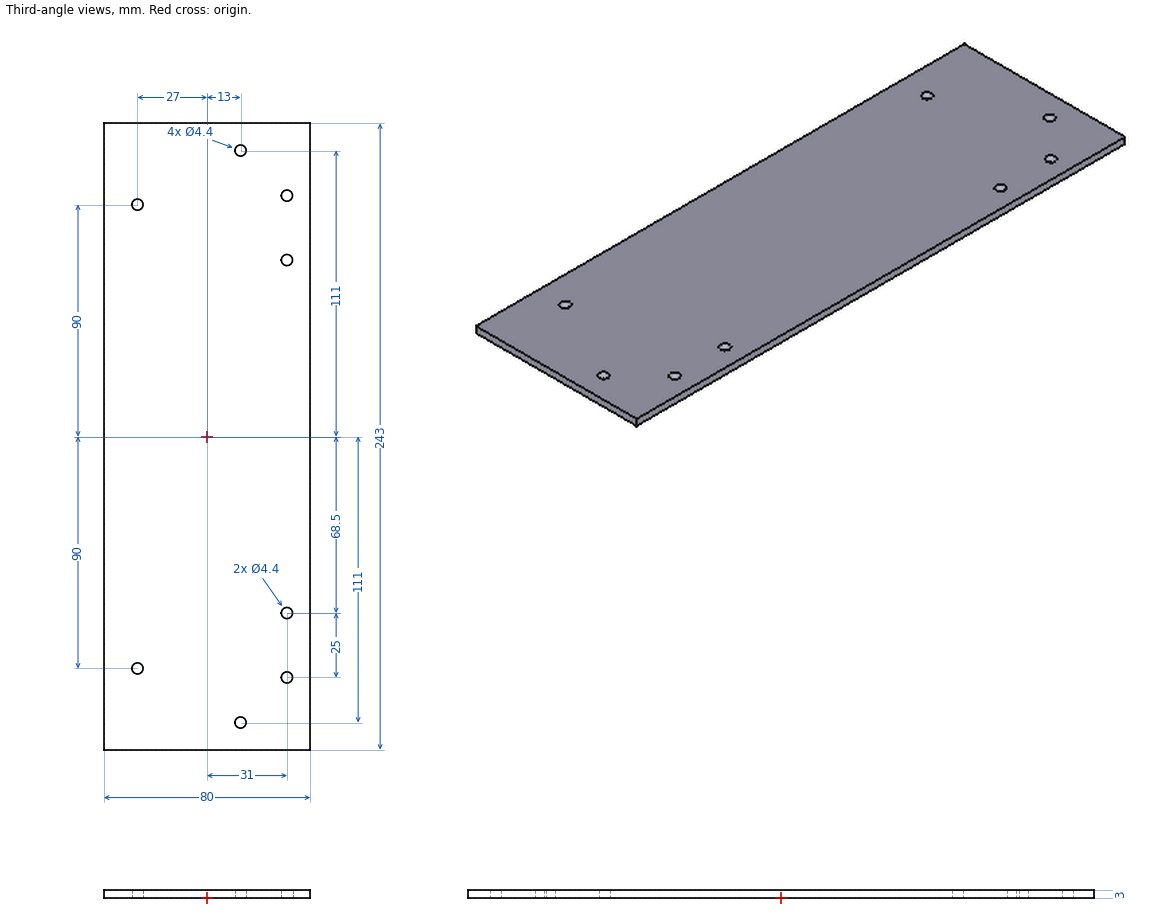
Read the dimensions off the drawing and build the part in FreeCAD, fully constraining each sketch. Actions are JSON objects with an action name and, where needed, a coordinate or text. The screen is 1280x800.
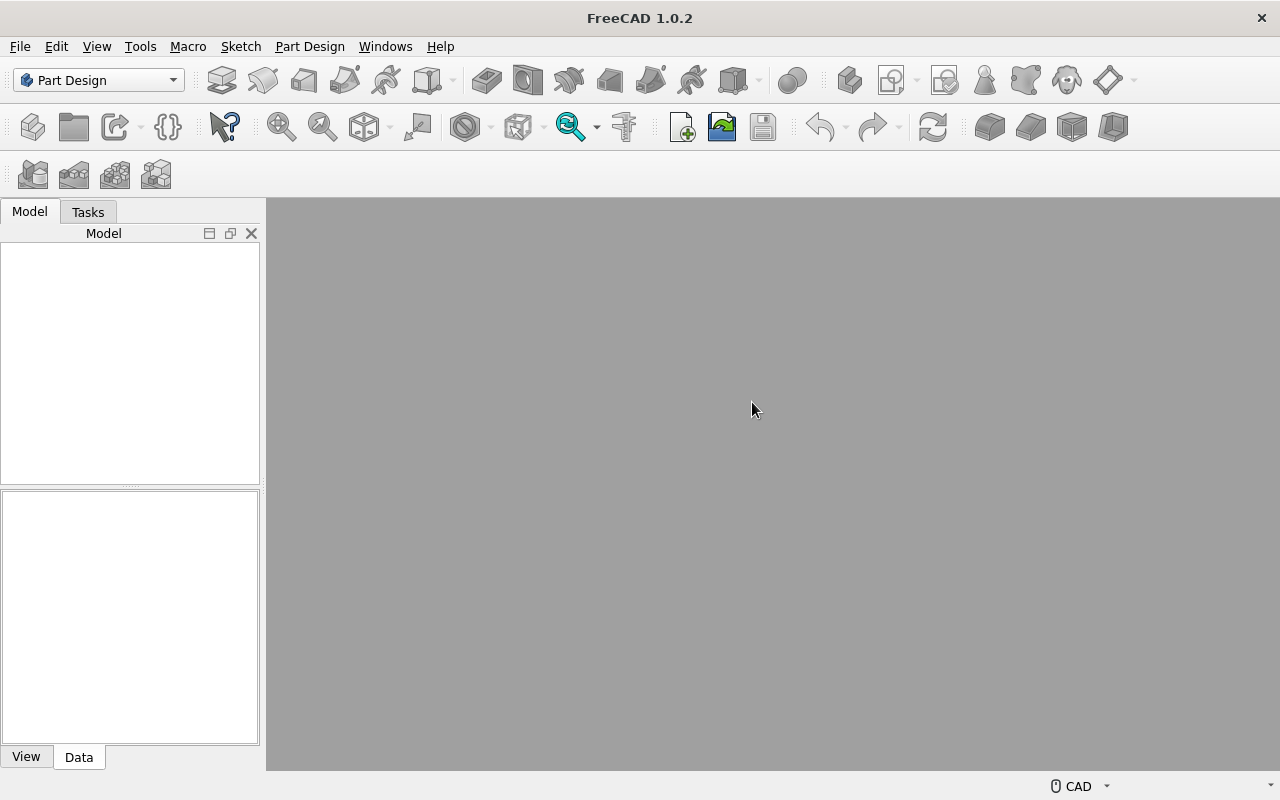
{"action": "left_click", "coordinate": [681, 128]}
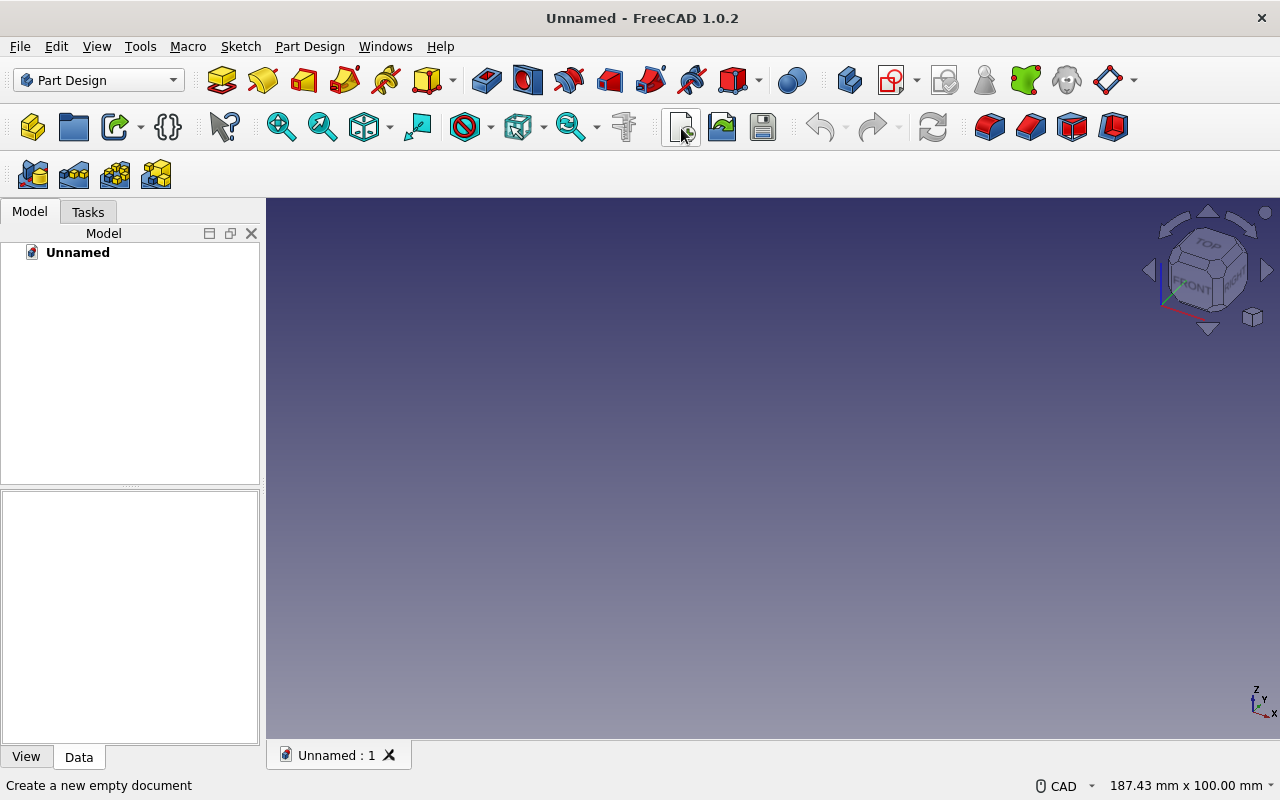
{"action": "left_click", "coordinate": [890, 80]}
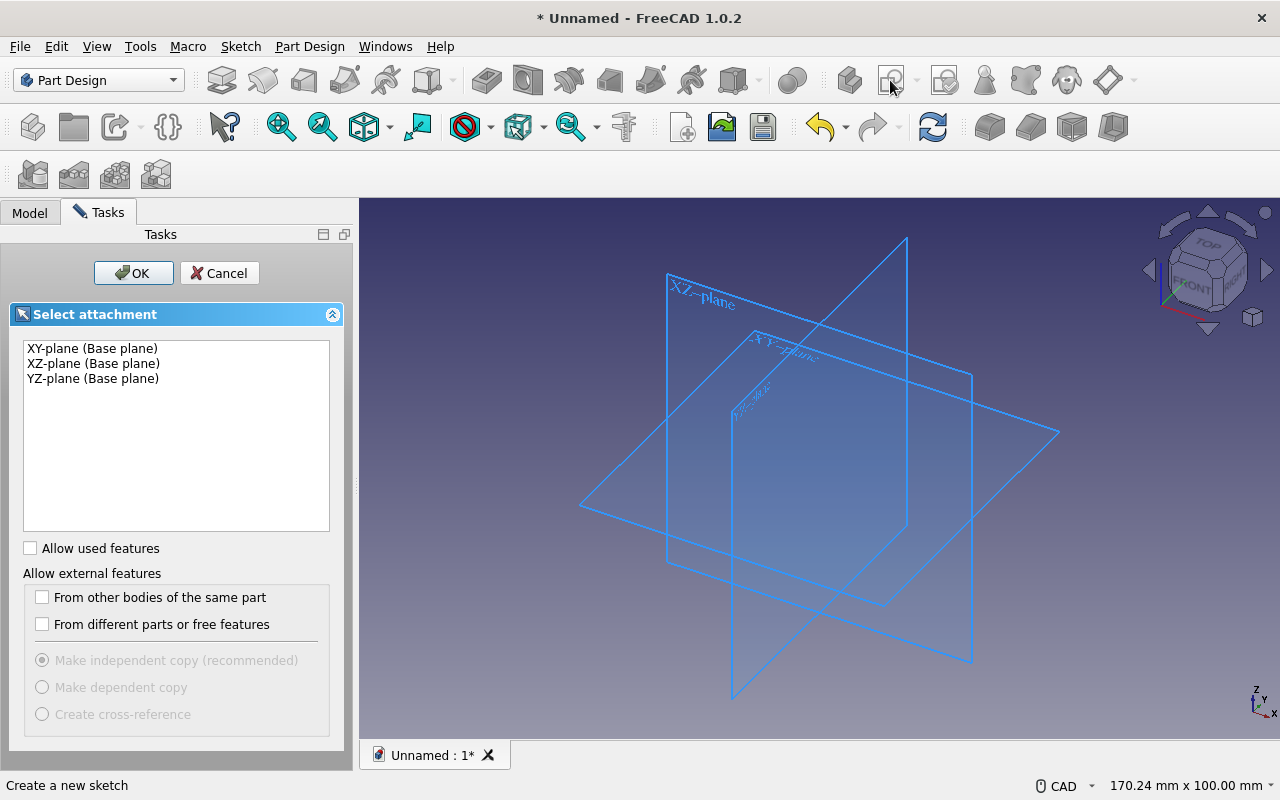
{"action": "left_click", "coordinate": [84, 348]}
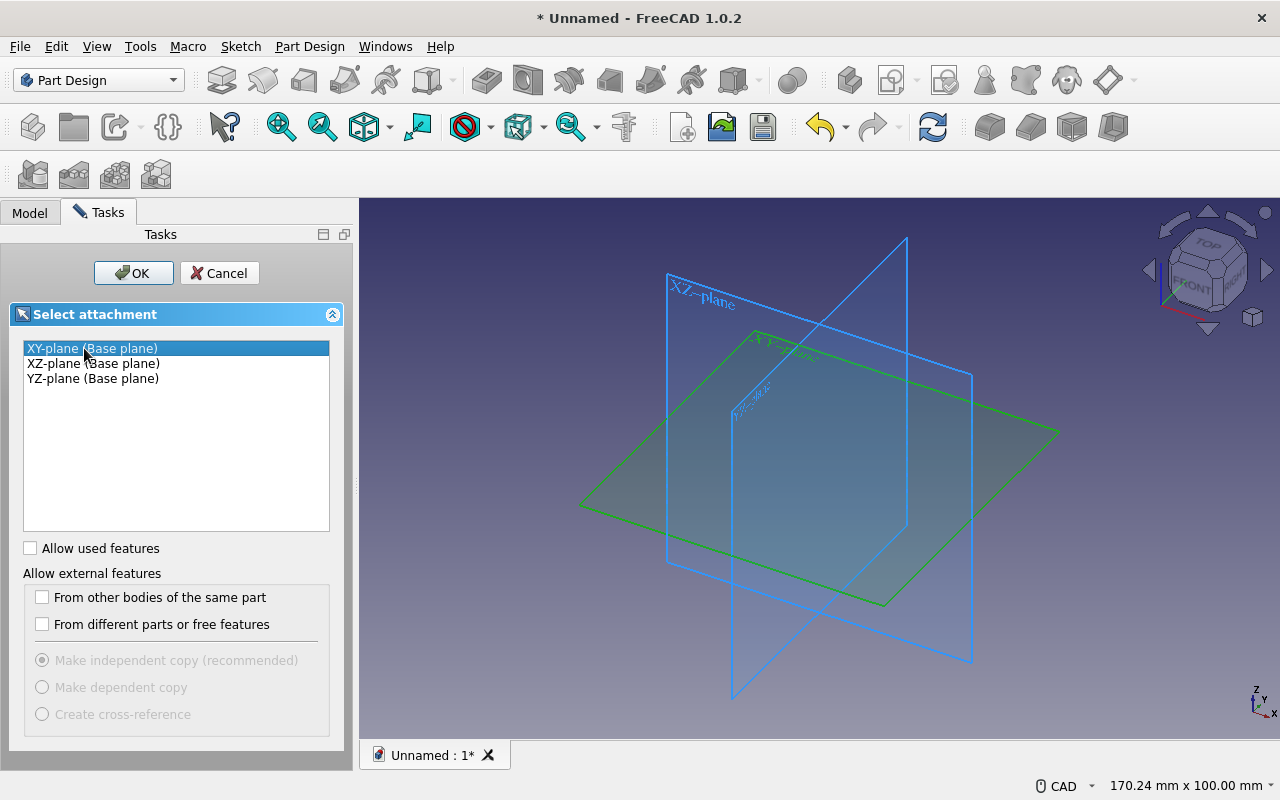
{"action": "left_click", "coordinate": [134, 273]}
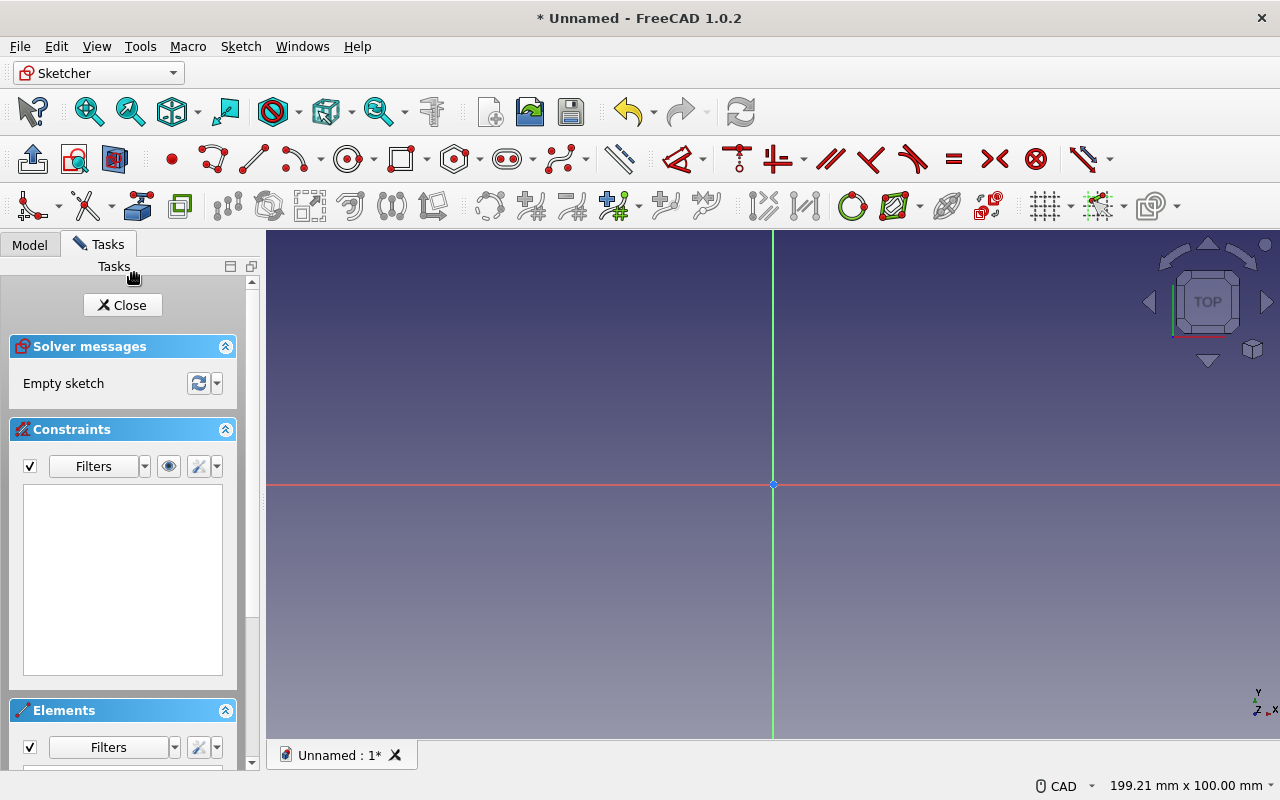
{"action": "scroll", "coordinate": [682, 485], "scroll_direction": "down", "scroll_amount": 7}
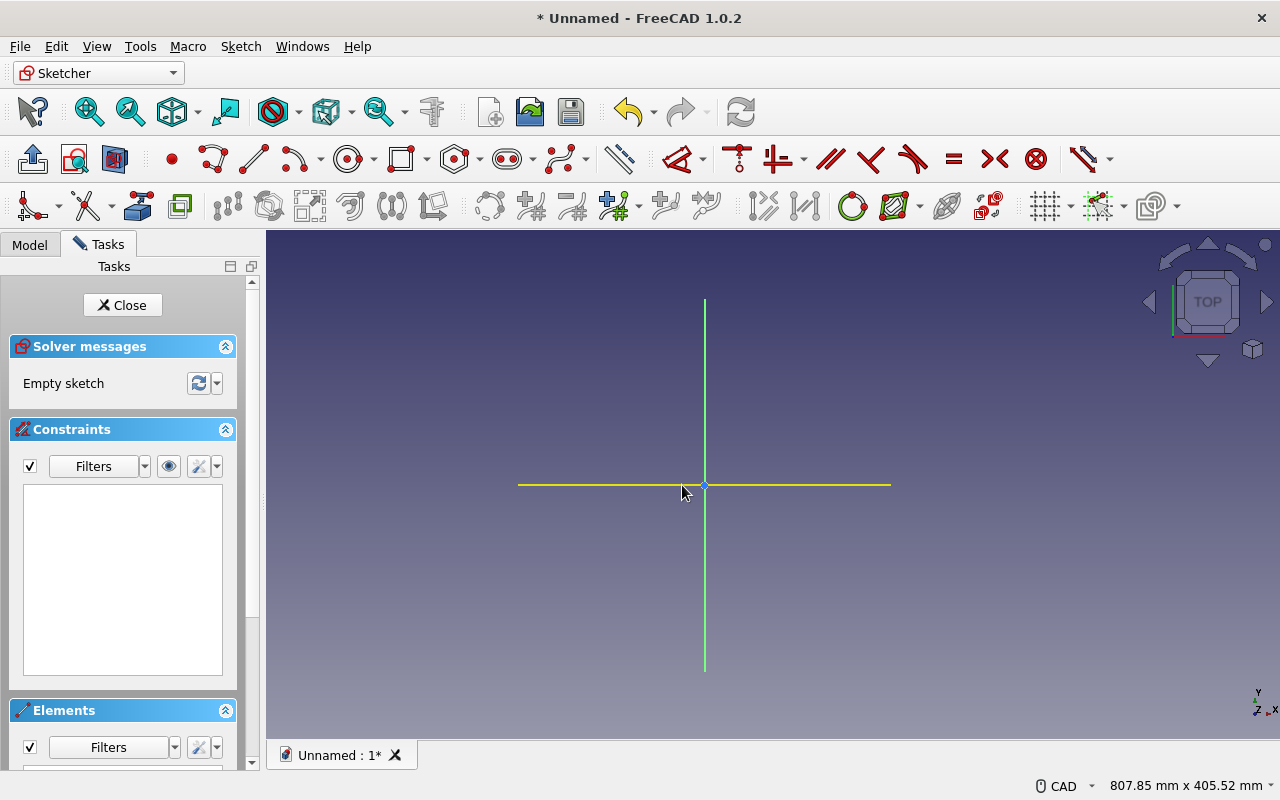
{"action": "left_click", "coordinate": [426, 160]}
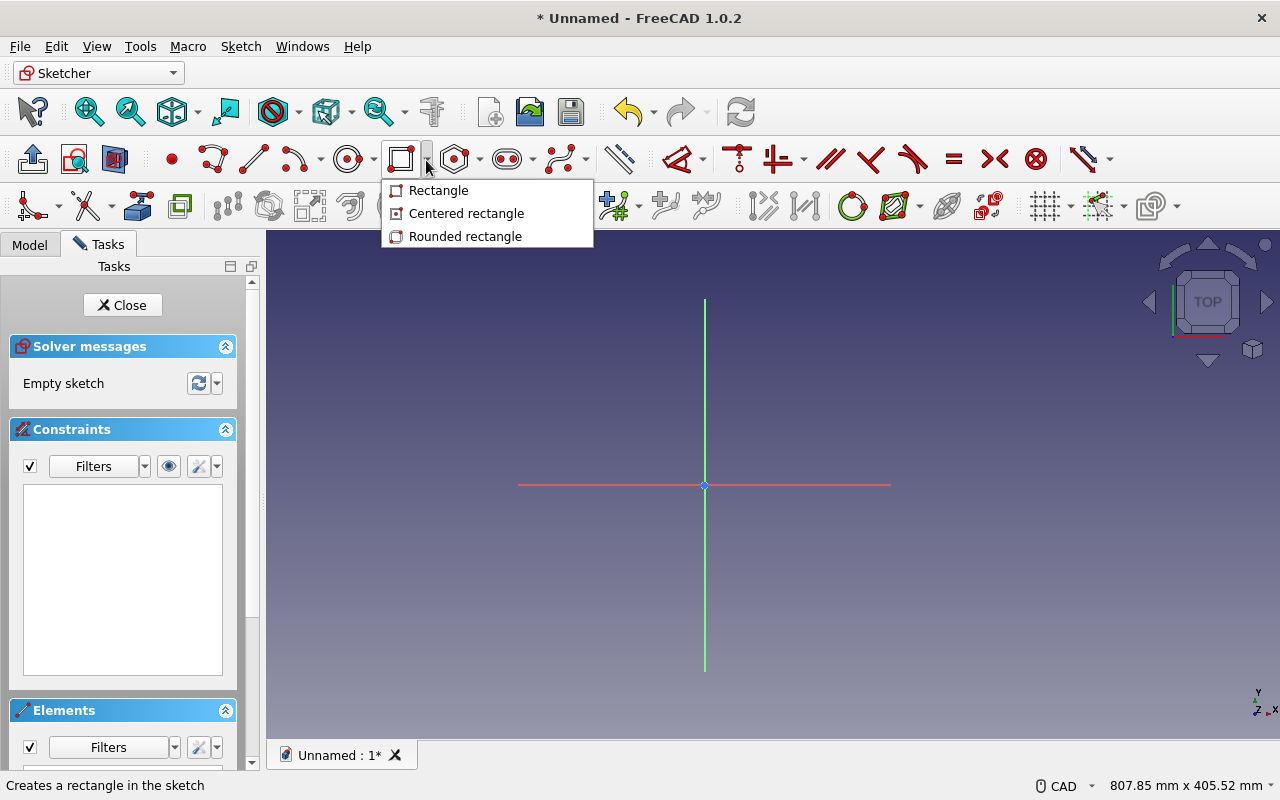
{"action": "left_click", "coordinate": [488, 214]}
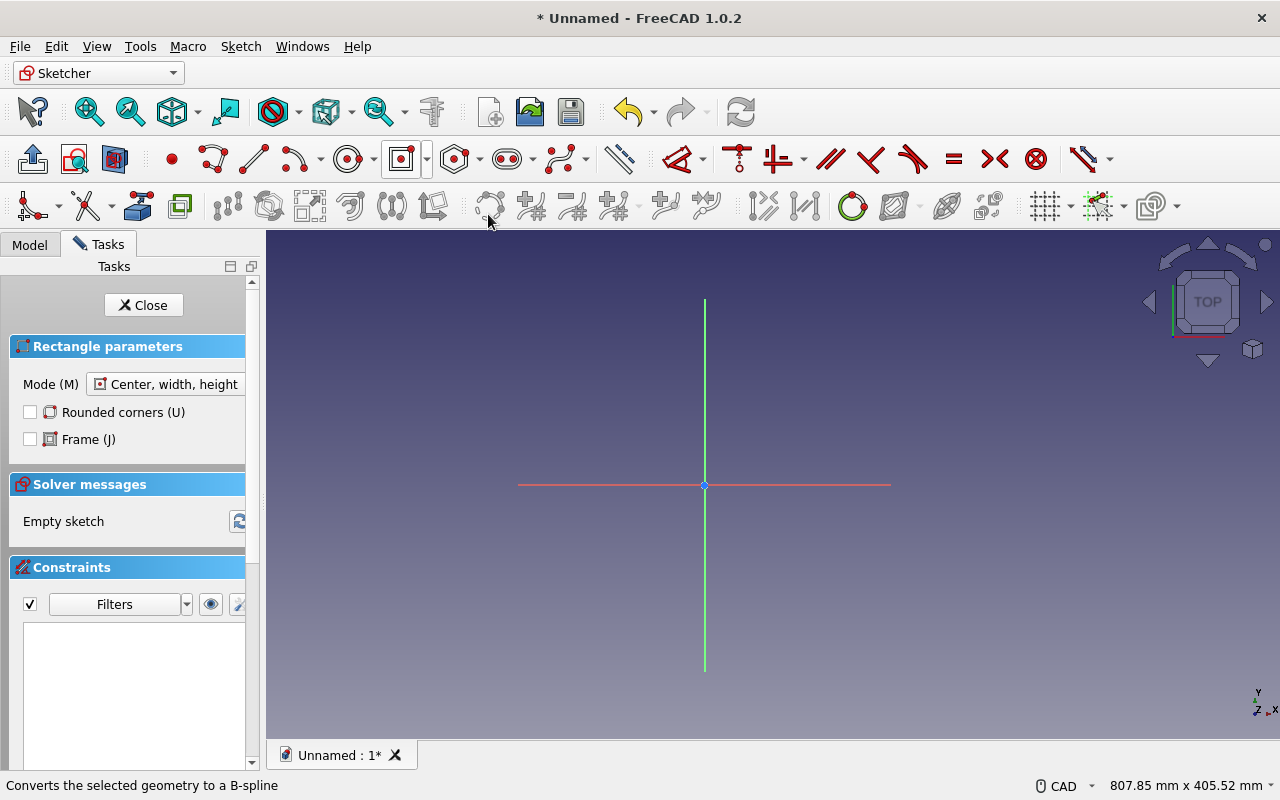
{"action": "left_click", "coordinate": [705, 485]}
{"action": "left_click", "coordinate": [755, 333]}
{"action": "key", "text": "Escape"}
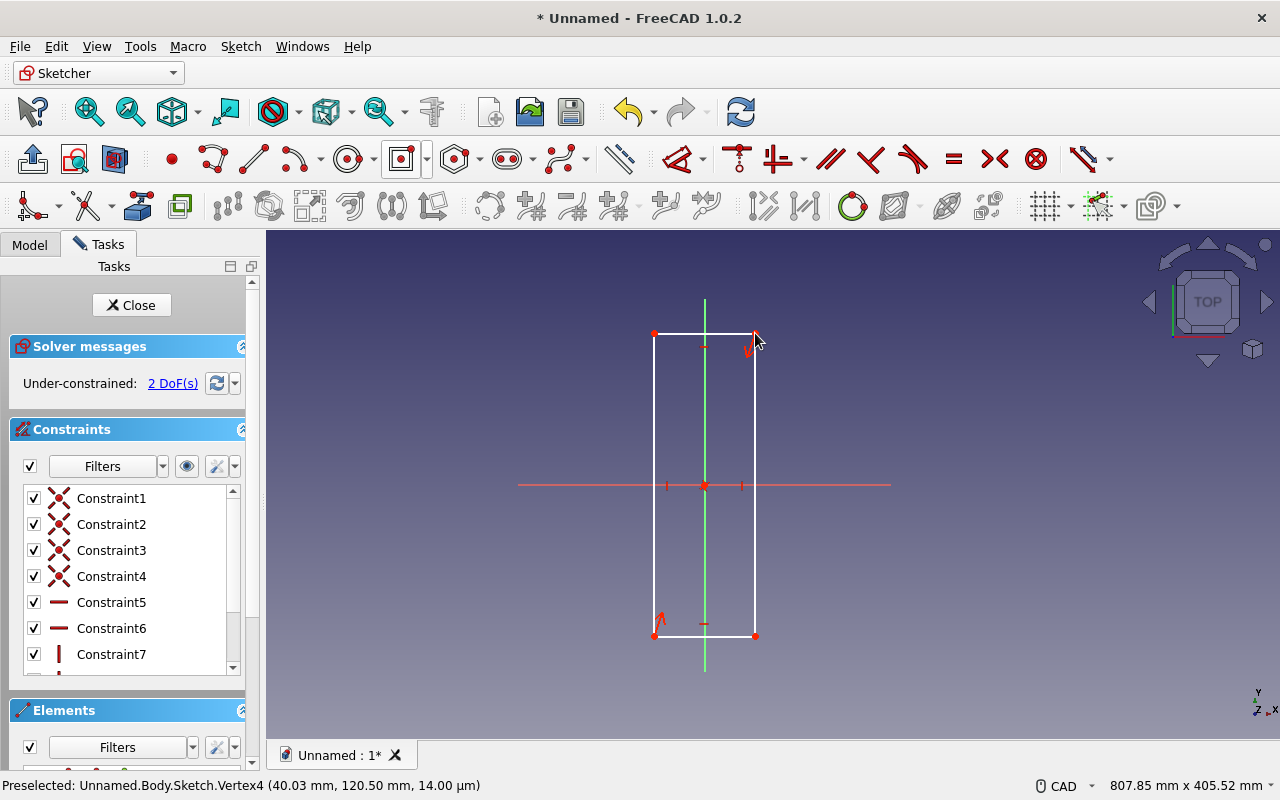
{"action": "left_click", "coordinate": [685, 637]}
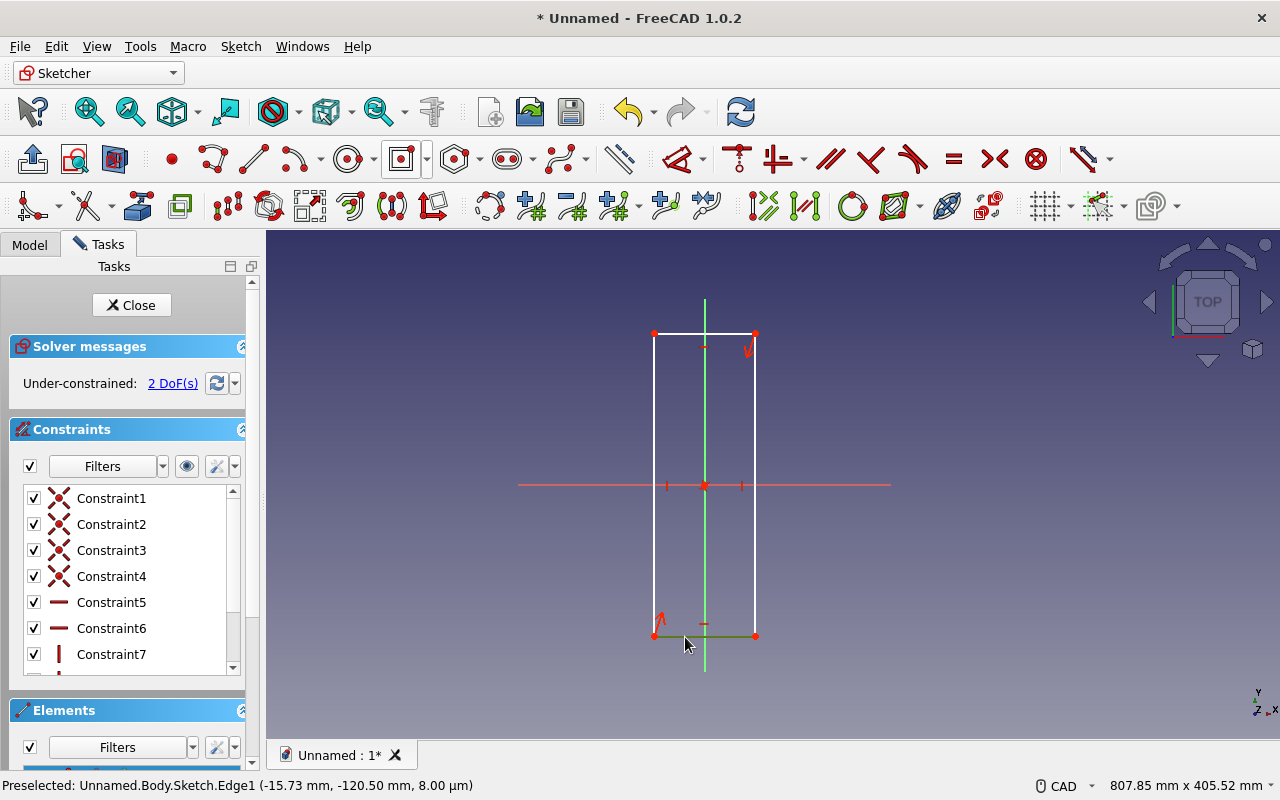
{"action": "left_click", "coordinate": [702, 160]}